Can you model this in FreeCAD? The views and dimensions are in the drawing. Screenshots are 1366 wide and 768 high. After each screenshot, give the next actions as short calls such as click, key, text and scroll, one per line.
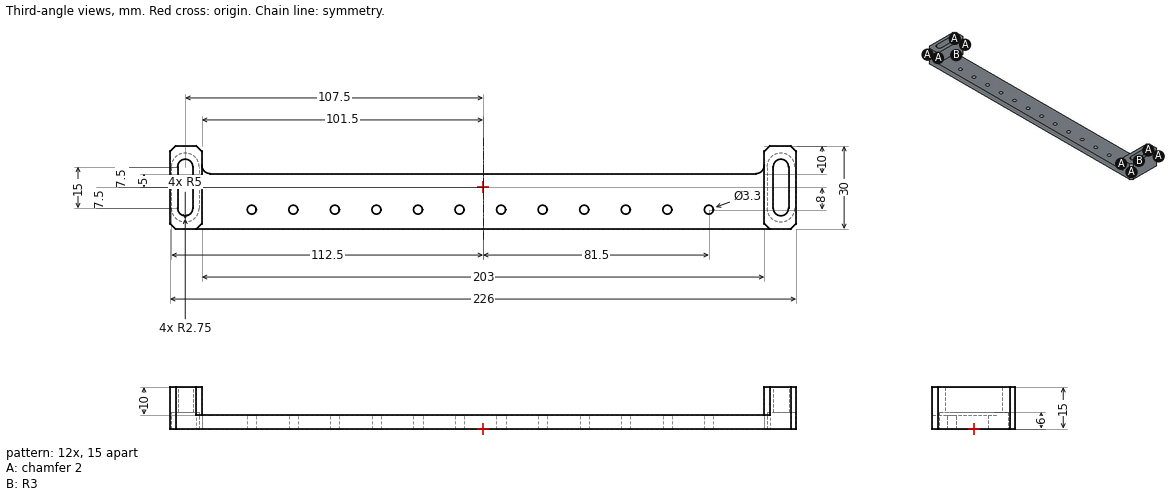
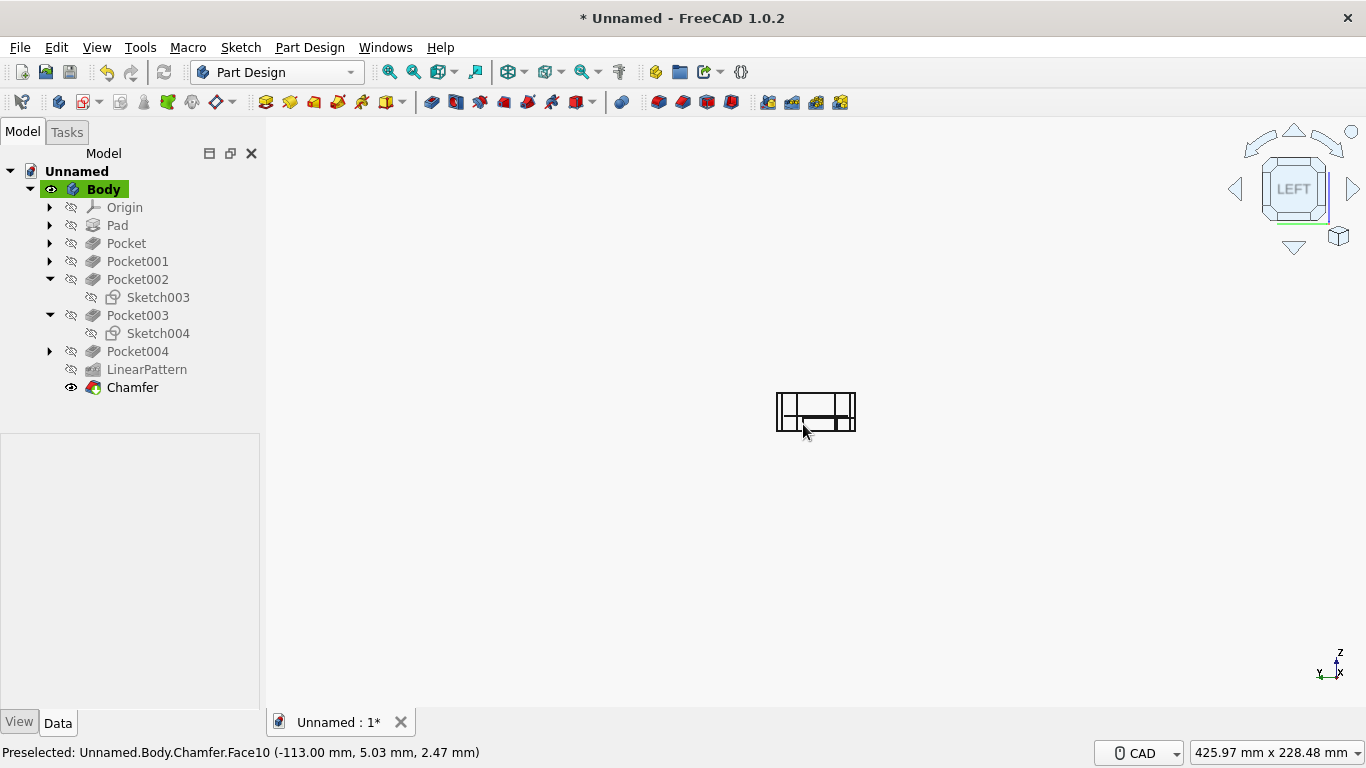
key(0)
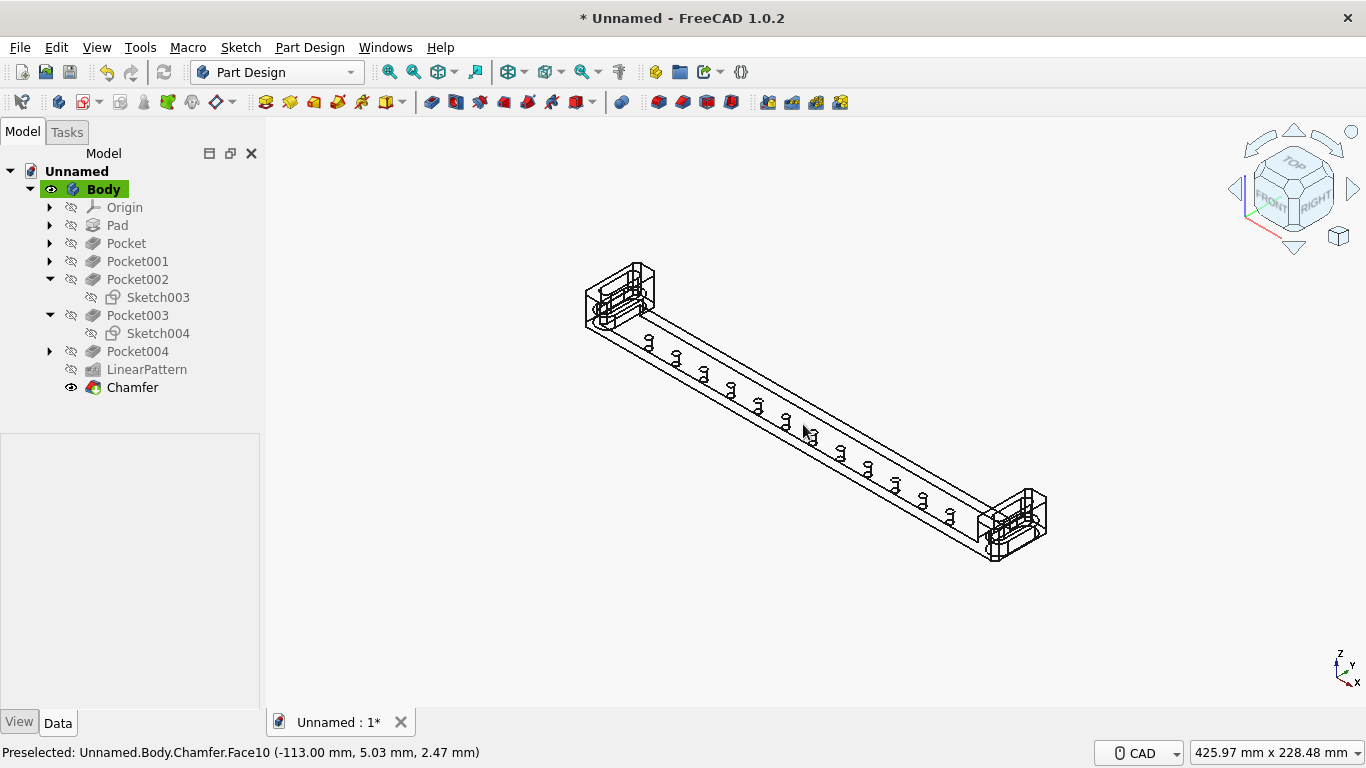
click(640, 312)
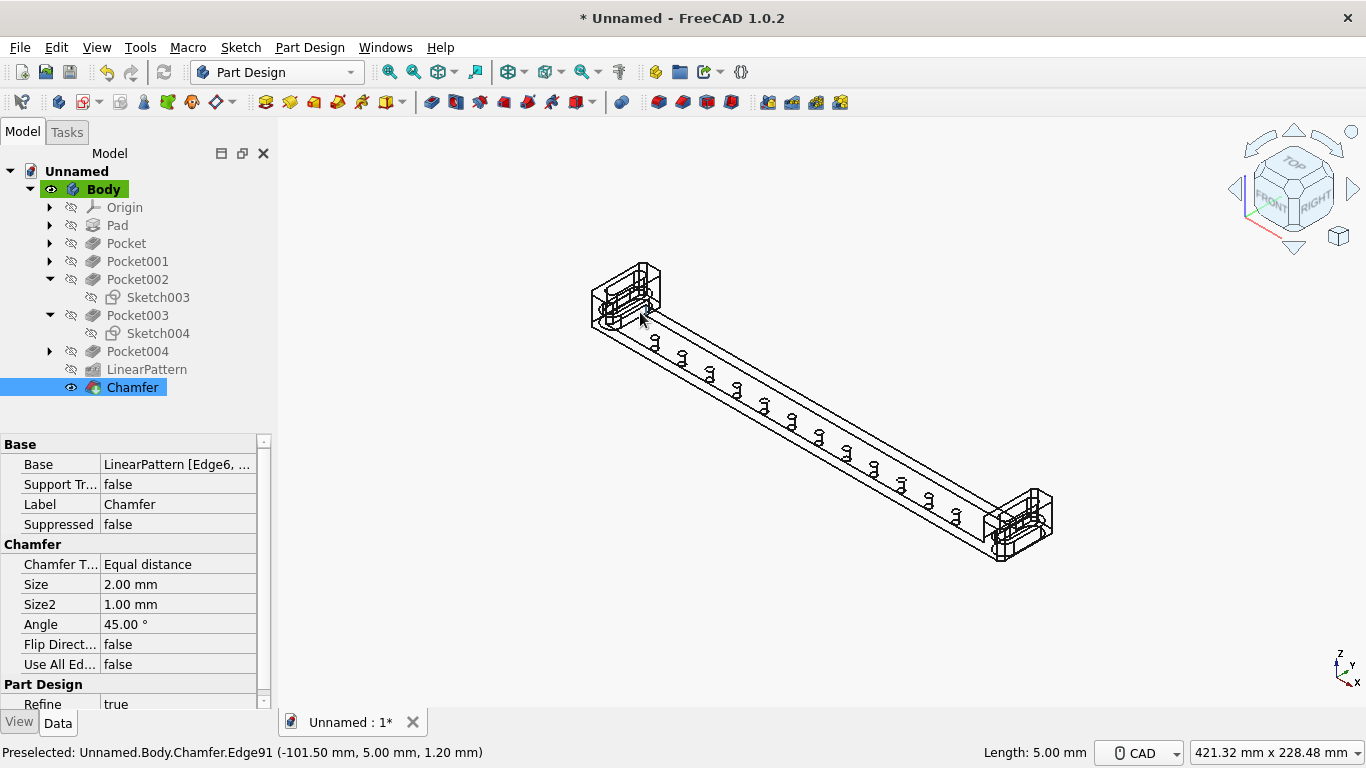
scroll(1016, 523, up, 6)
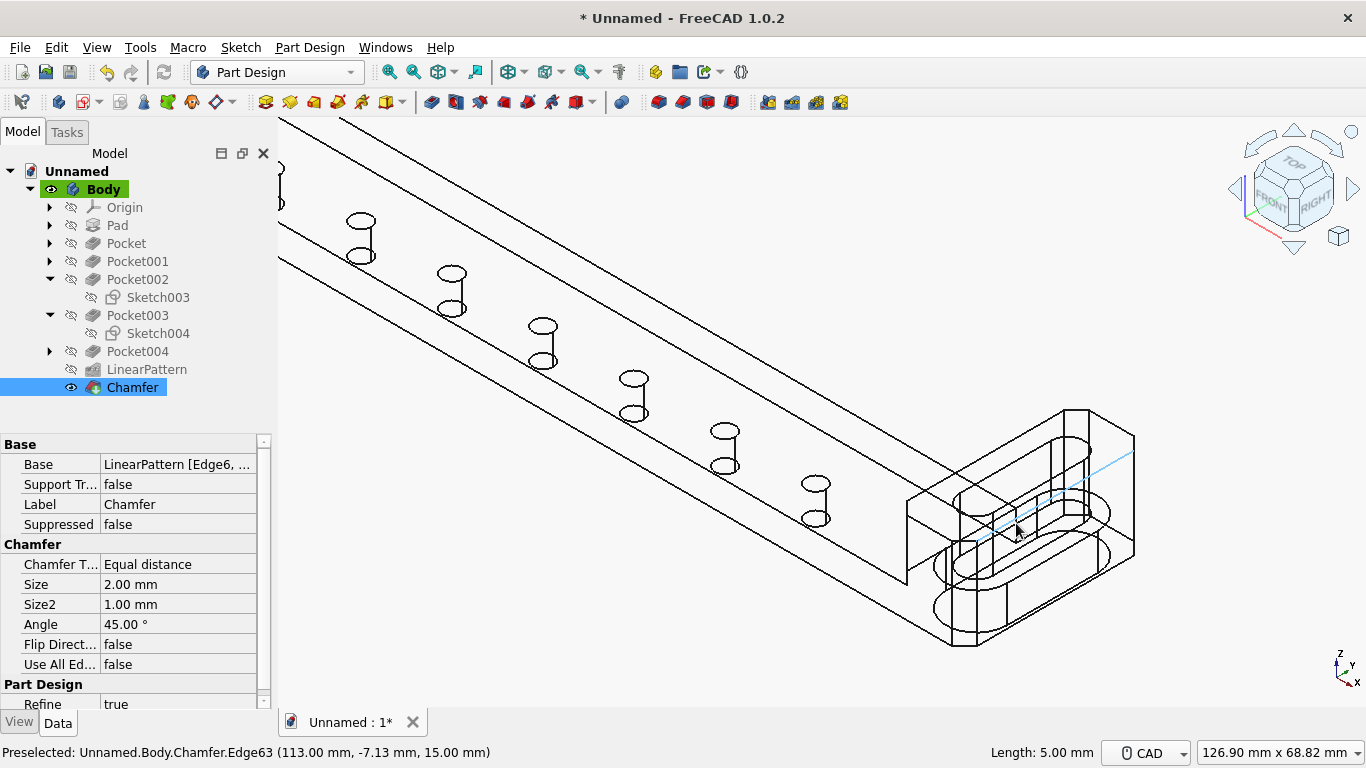
click(1016, 532, ctrl)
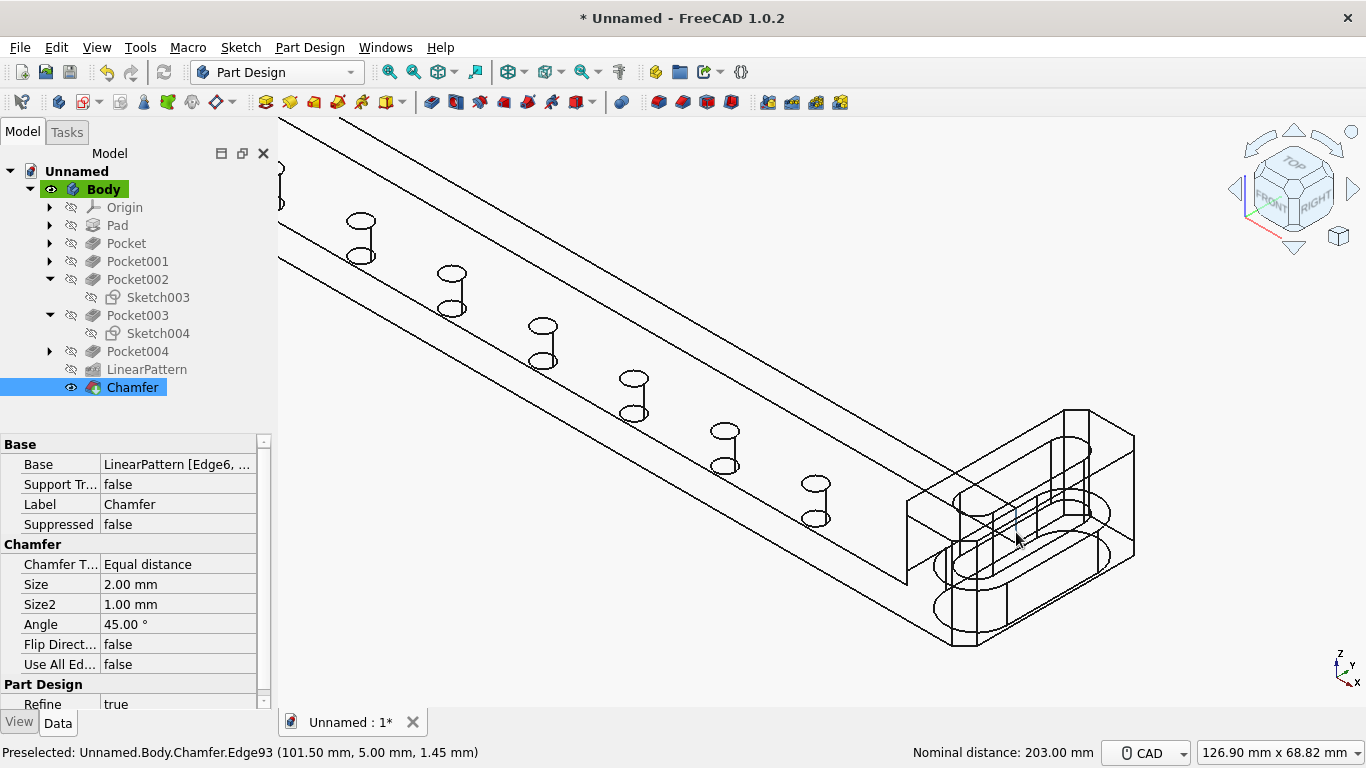
key(v)
key(1)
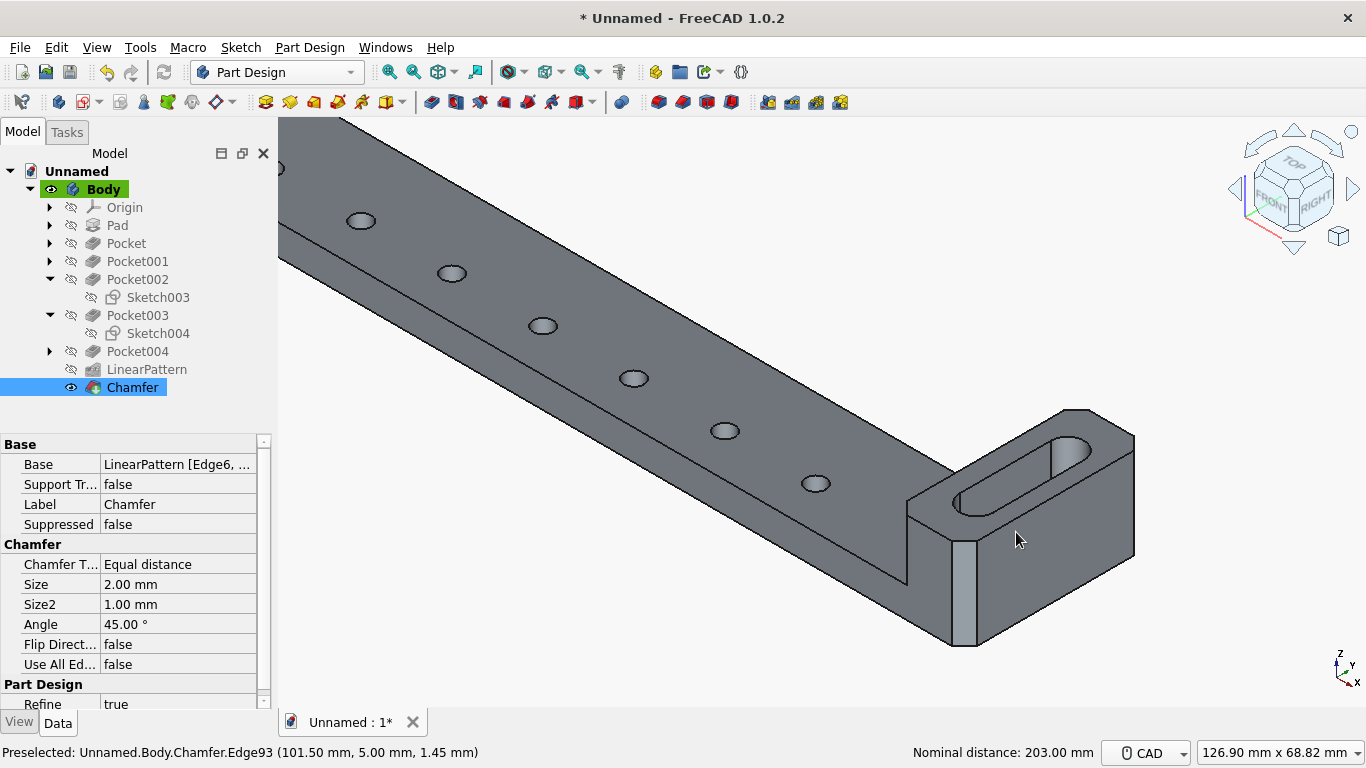
click(660, 102)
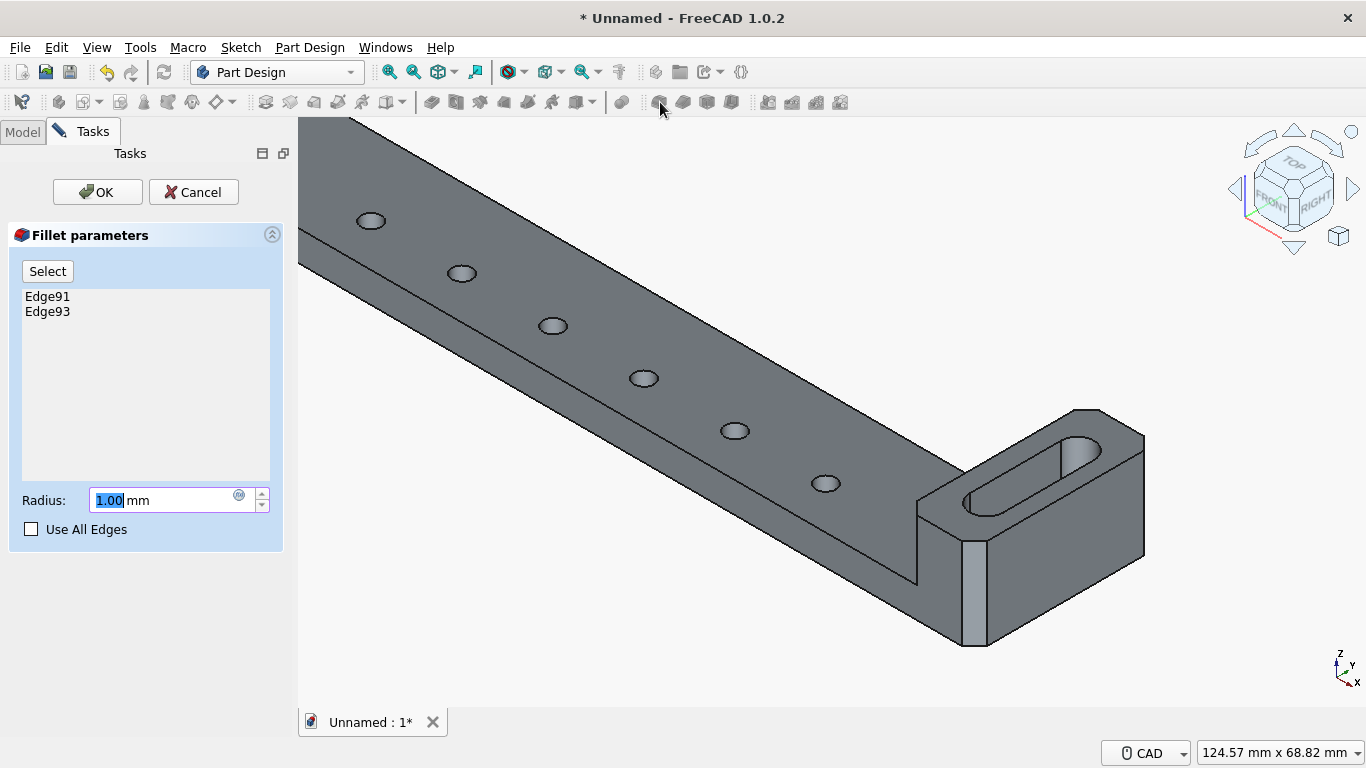
text(3)
key(Tab)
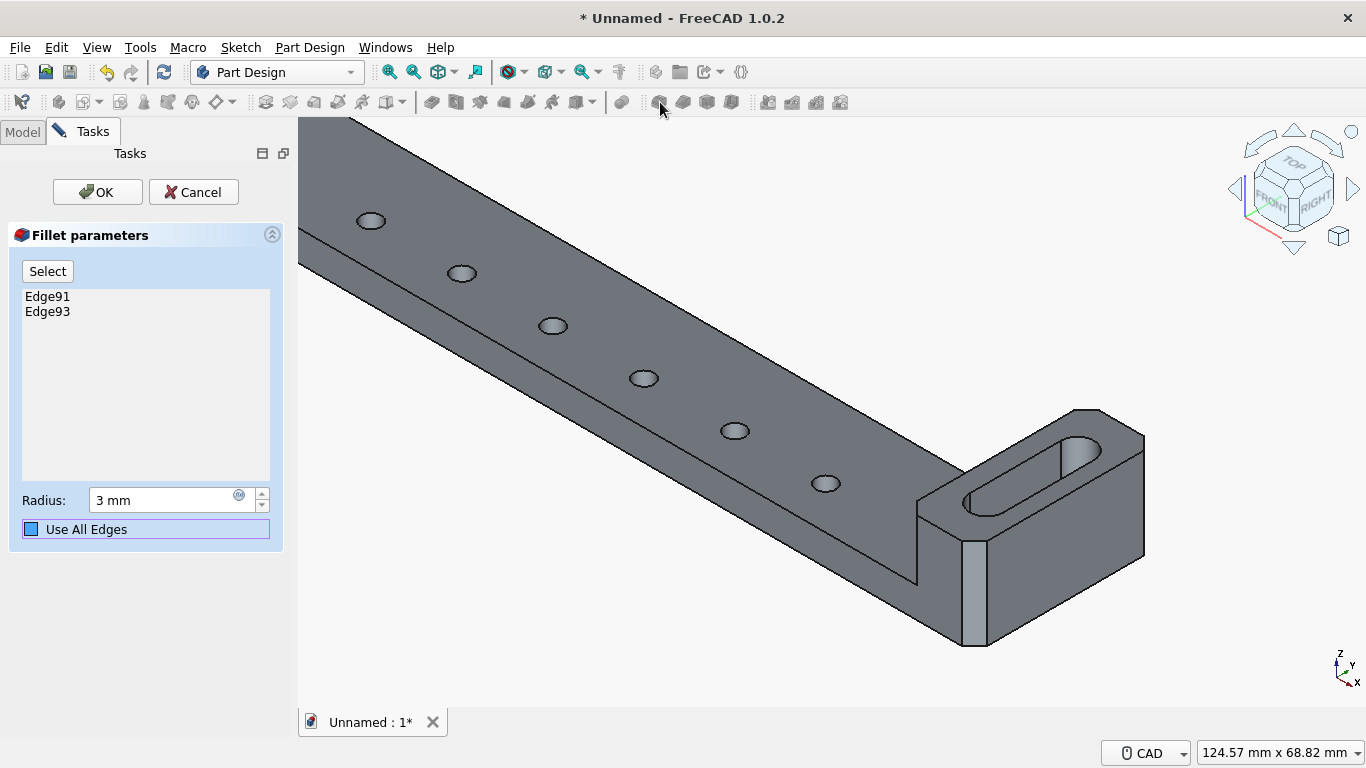
click(98, 192)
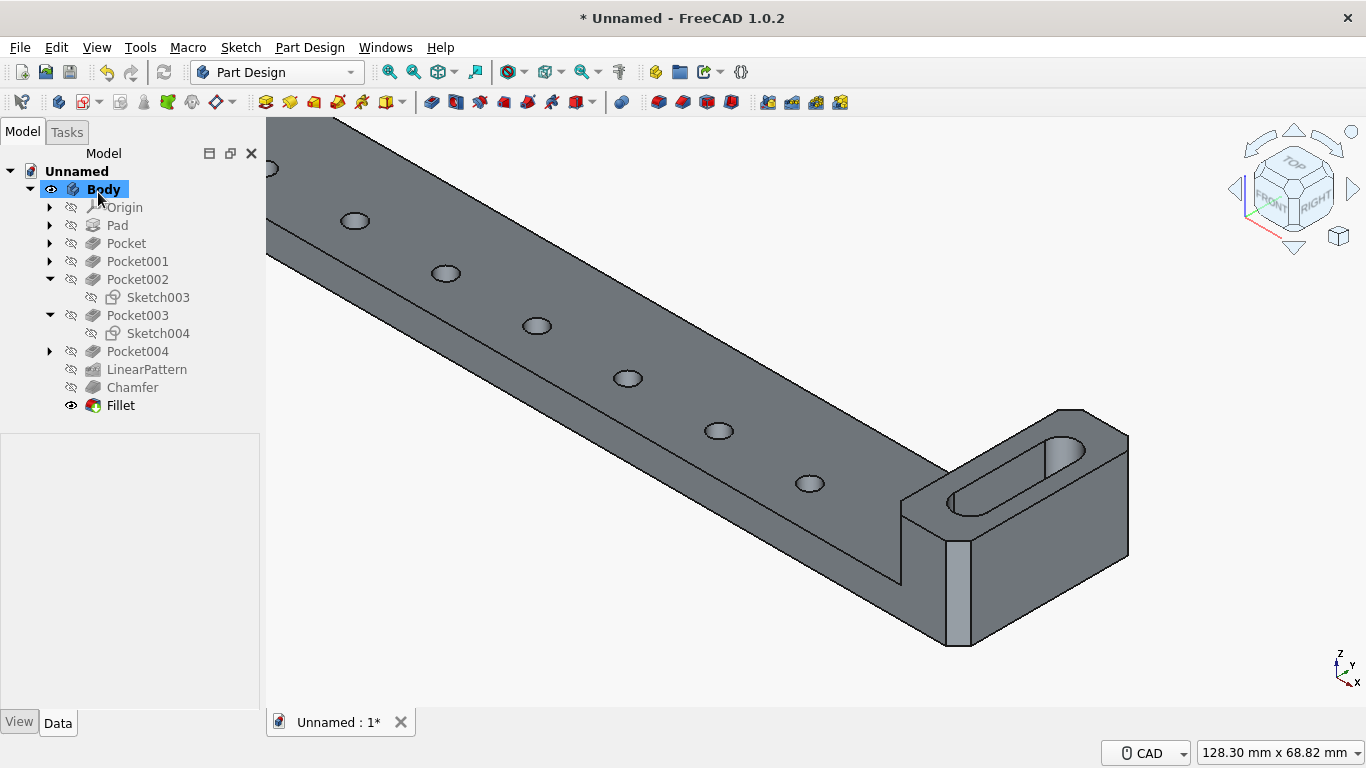
key(v)
key(f)